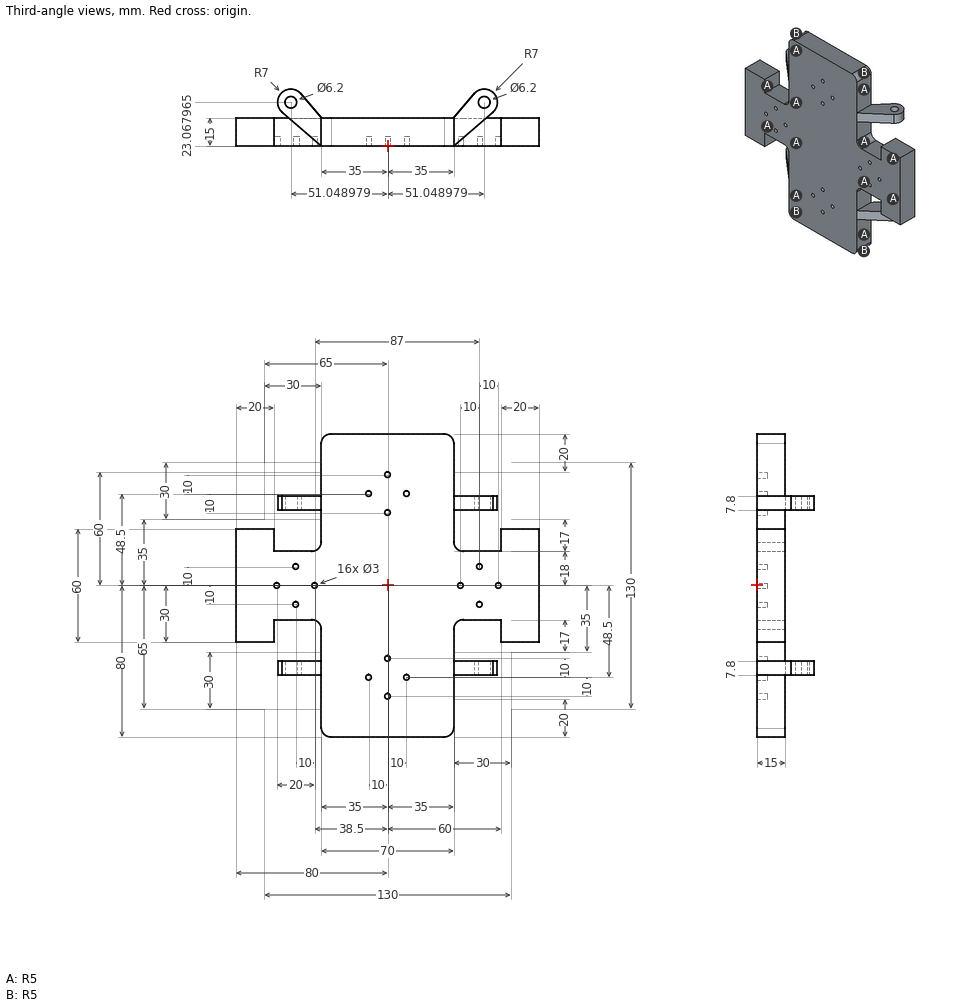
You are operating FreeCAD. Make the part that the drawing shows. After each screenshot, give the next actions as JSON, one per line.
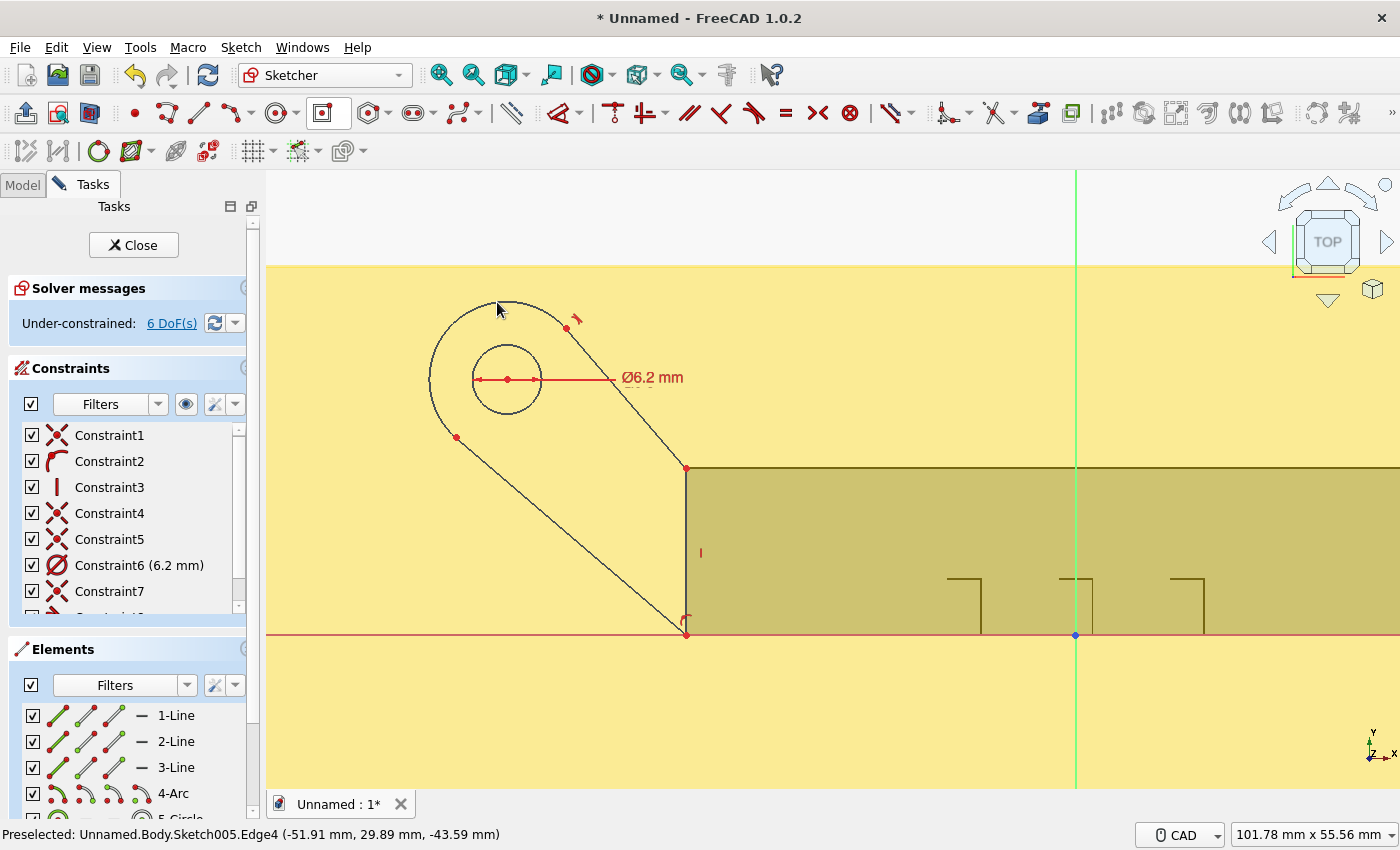
{"action": "left_click", "coordinate": [617, 576]}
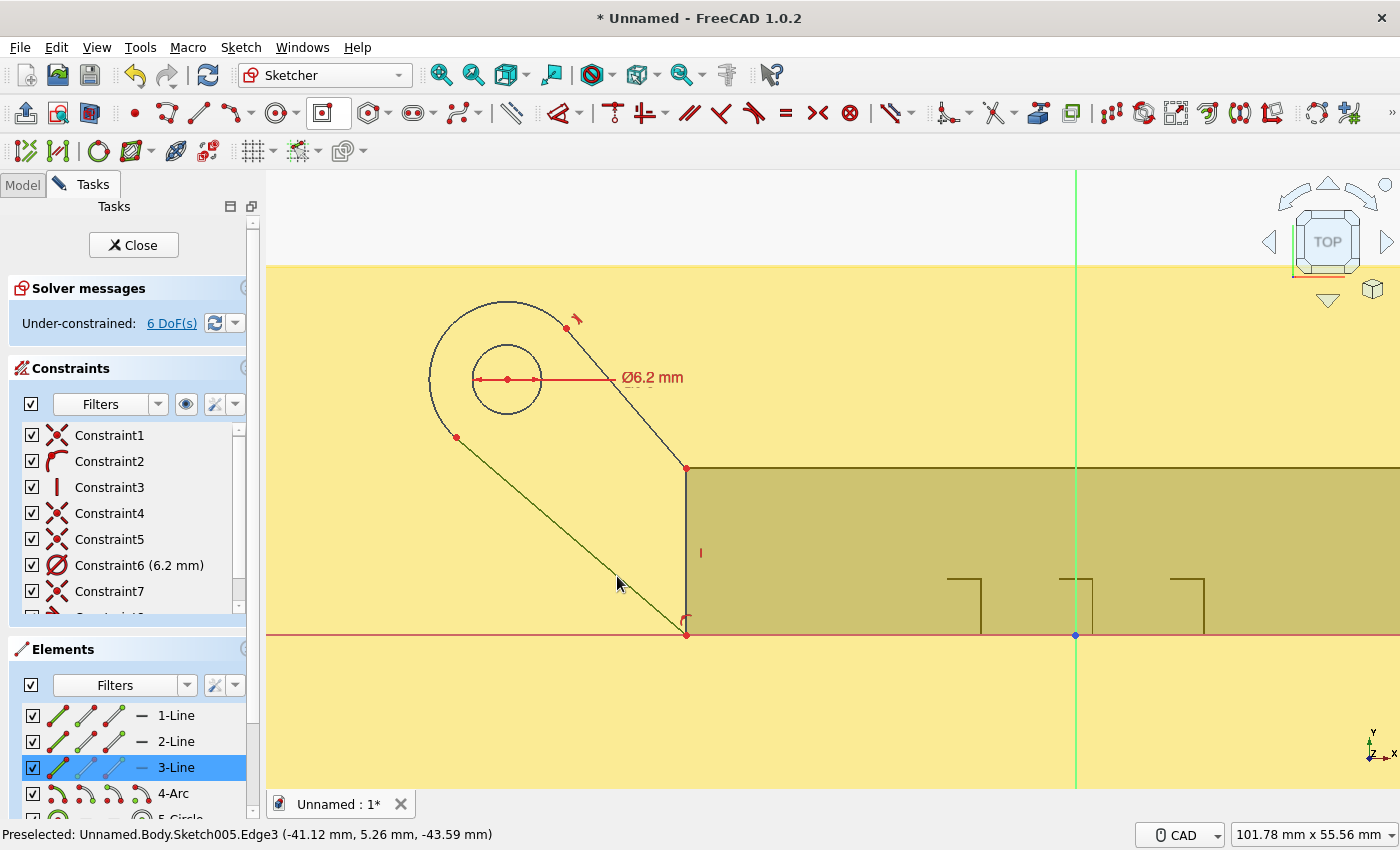
{"action": "left_click", "coordinate": [497, 302]}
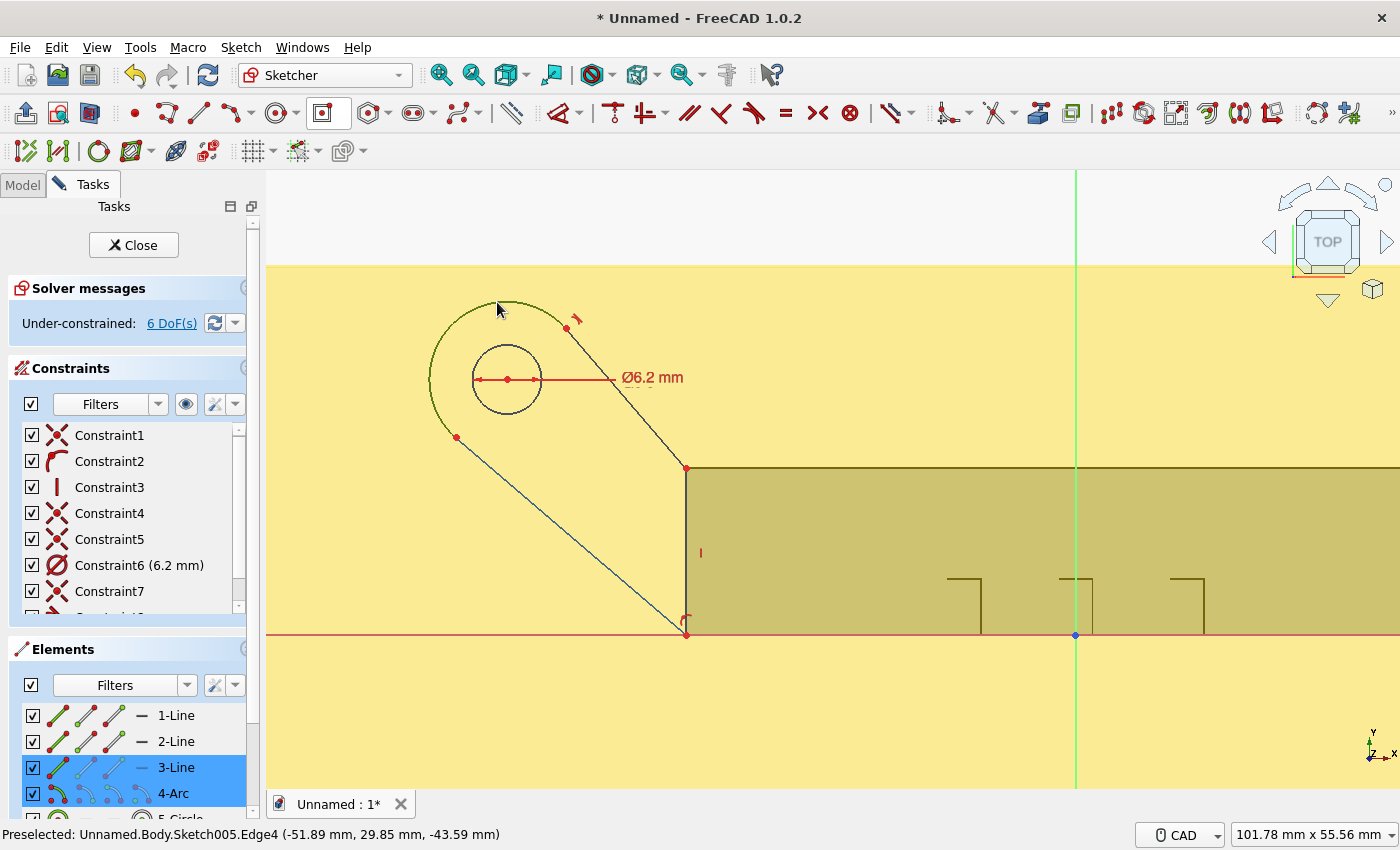
{"action": "left_click", "coordinate": [754, 114]}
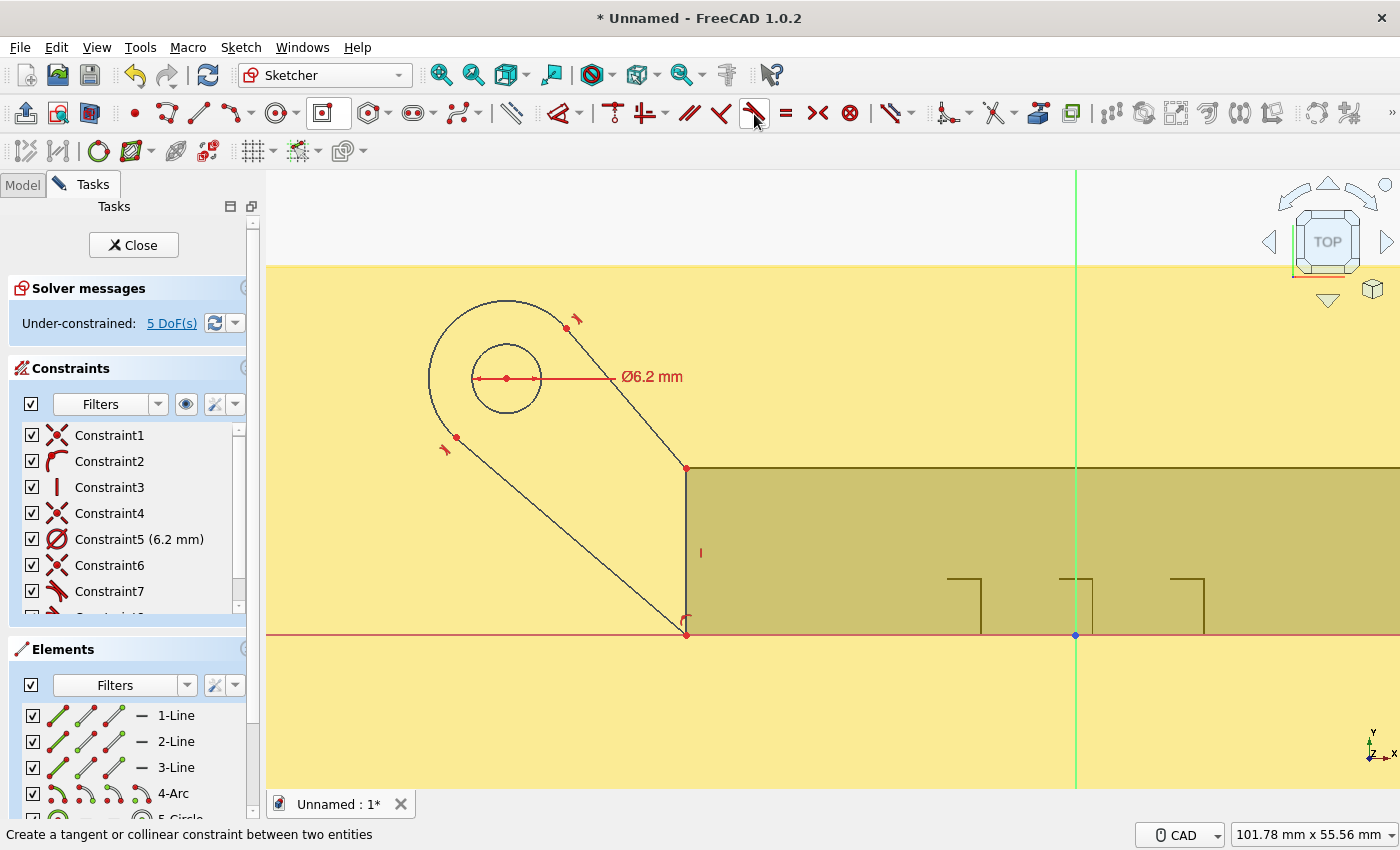
{"action": "left_click", "coordinate": [558, 114]}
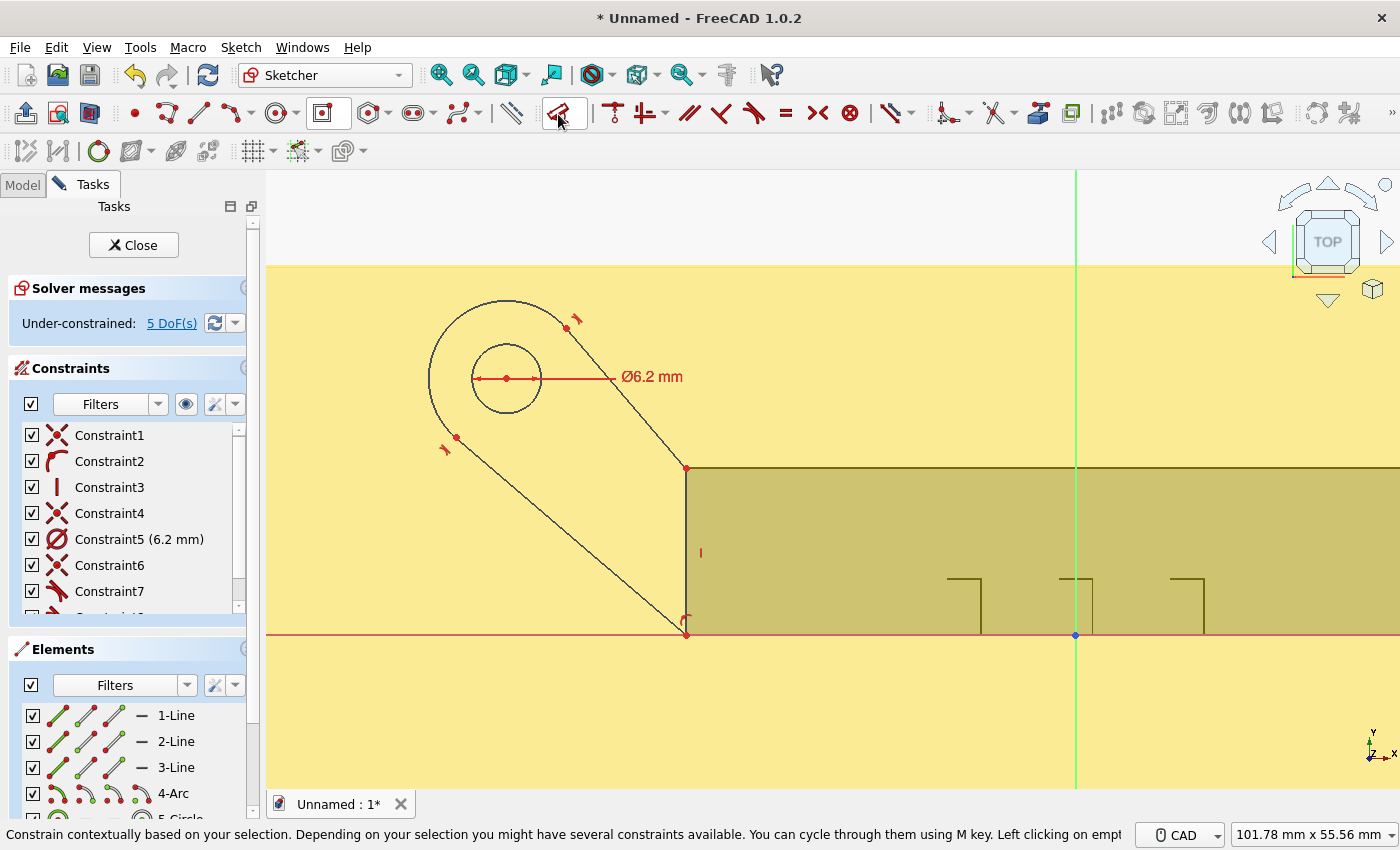
{"action": "left_click", "coordinate": [497, 301]}
{"action": "left_click", "coordinate": [493, 269]}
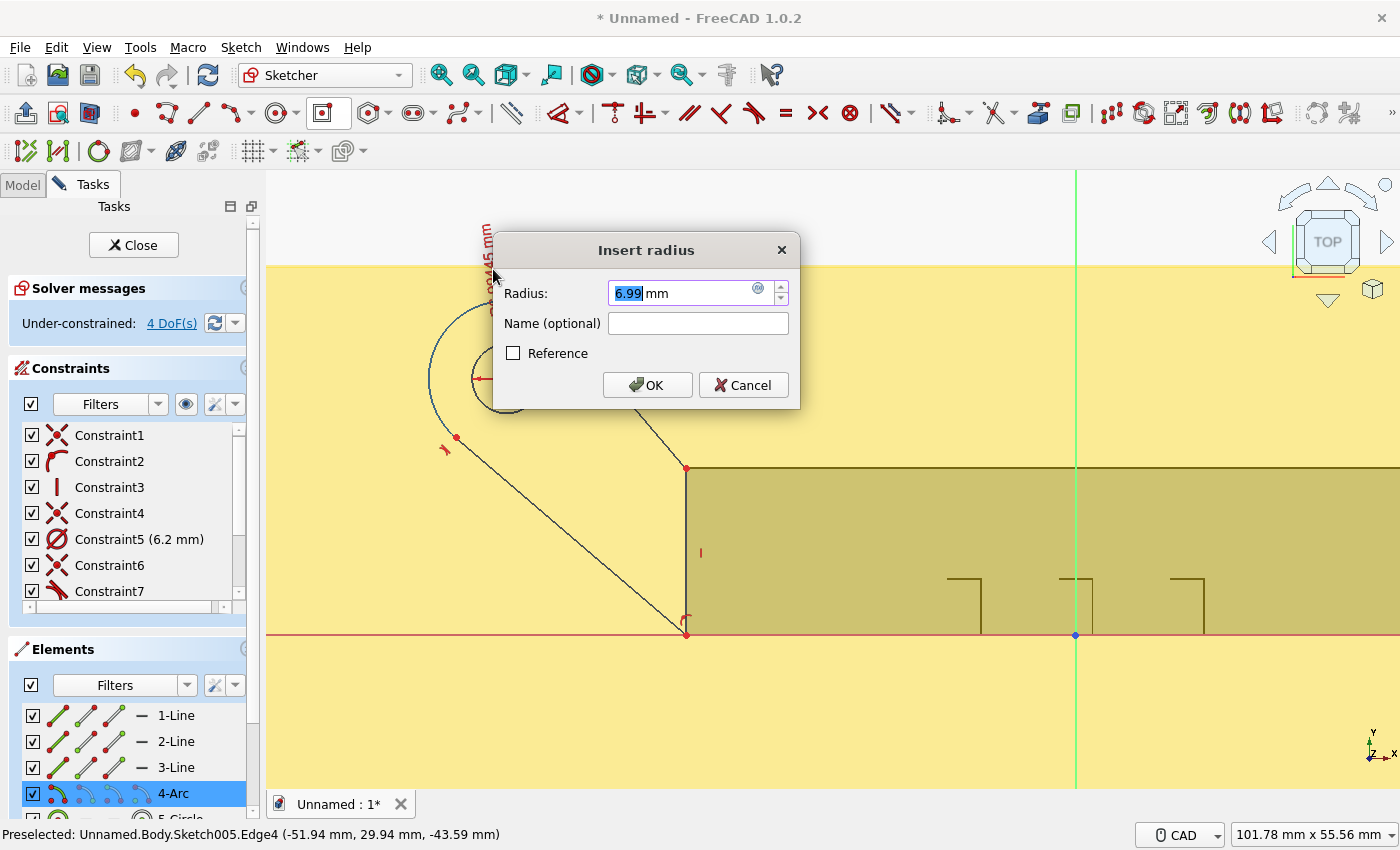
{"action": "type", "text": "7"}
{"action": "key", "text": "Return"}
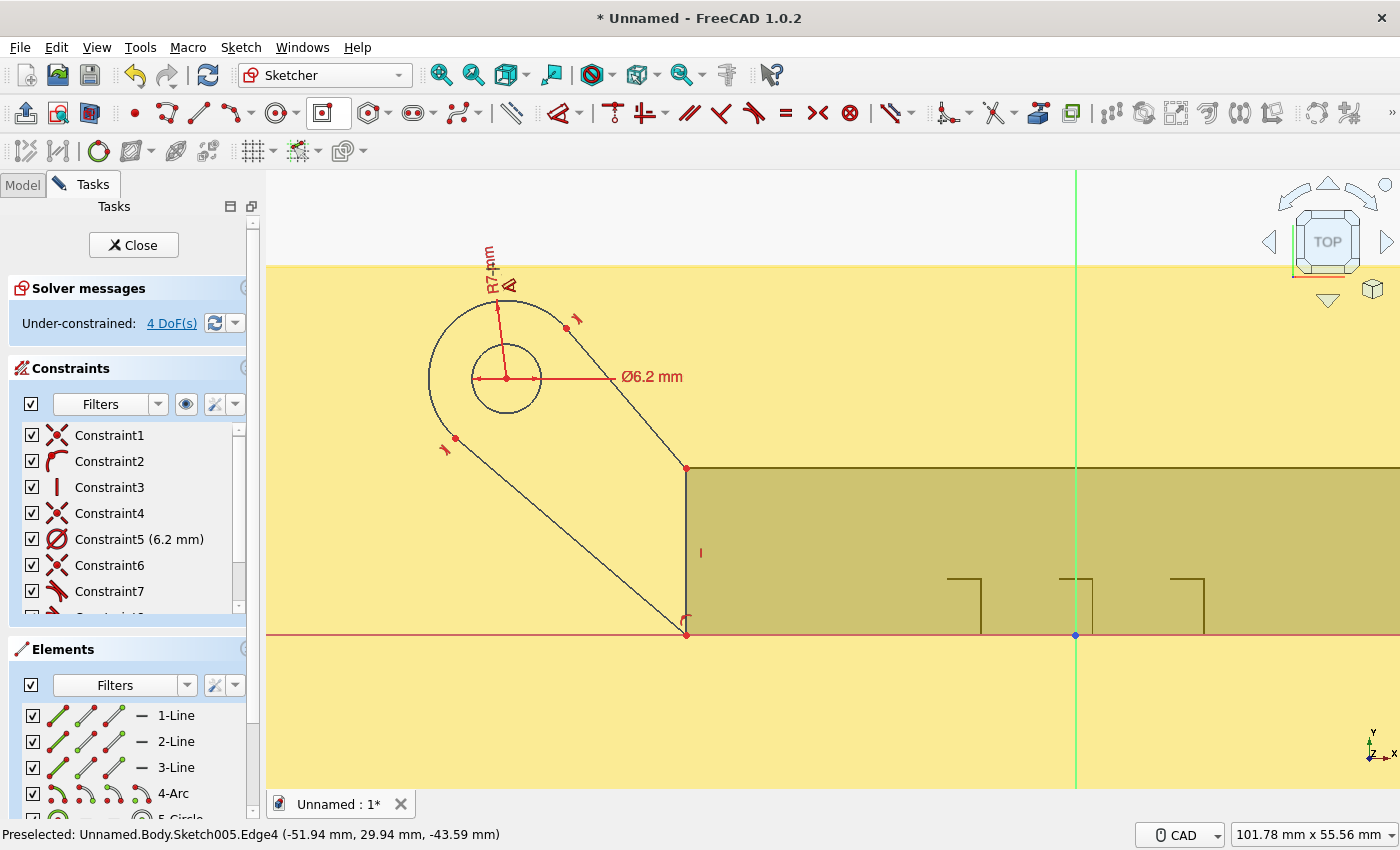
{"action": "left_click", "coordinate": [686, 519]}
{"action": "left_click", "coordinate": [652, 552]}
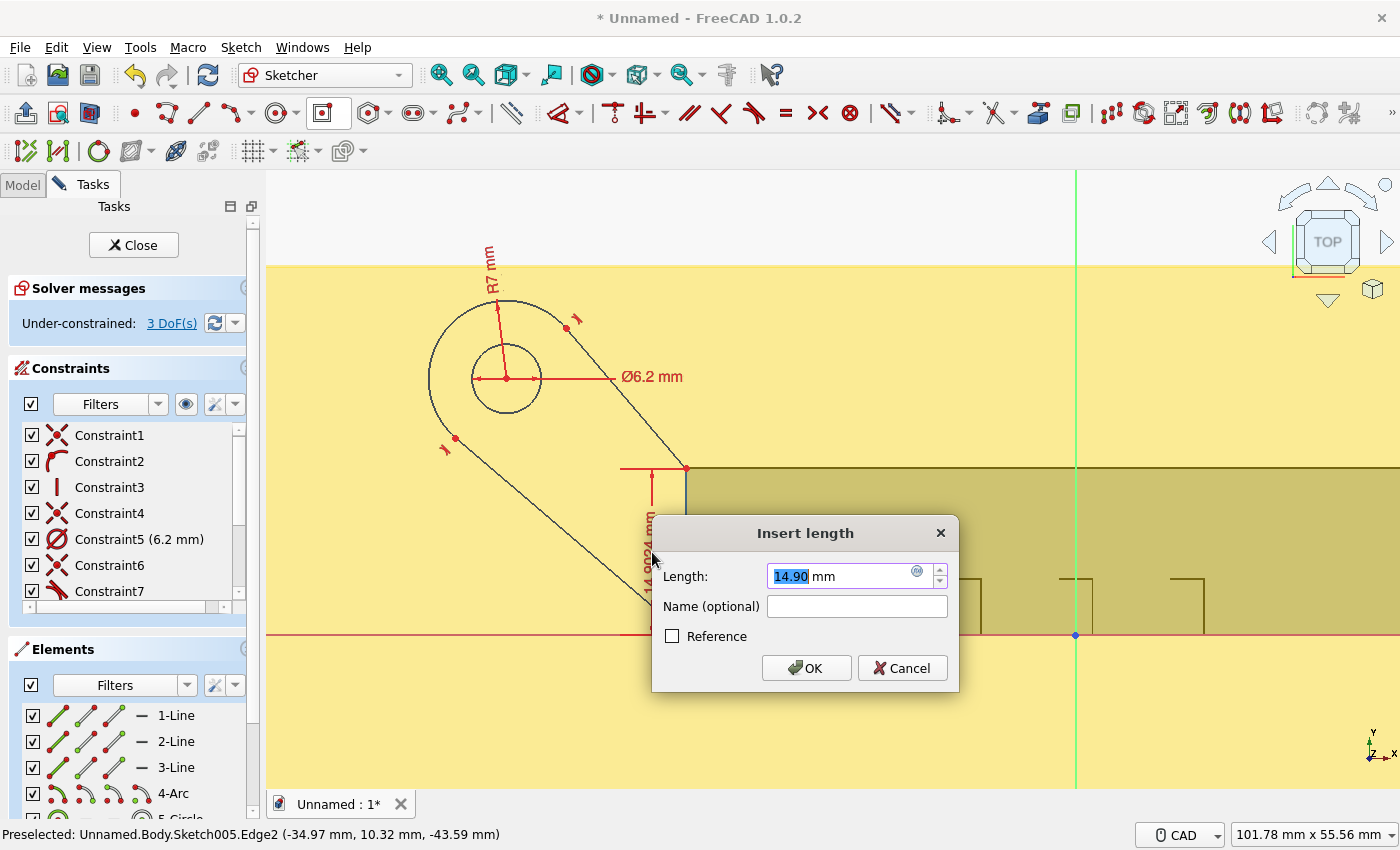
{"action": "type", "text": "15"}
{"action": "key", "text": "Return"}